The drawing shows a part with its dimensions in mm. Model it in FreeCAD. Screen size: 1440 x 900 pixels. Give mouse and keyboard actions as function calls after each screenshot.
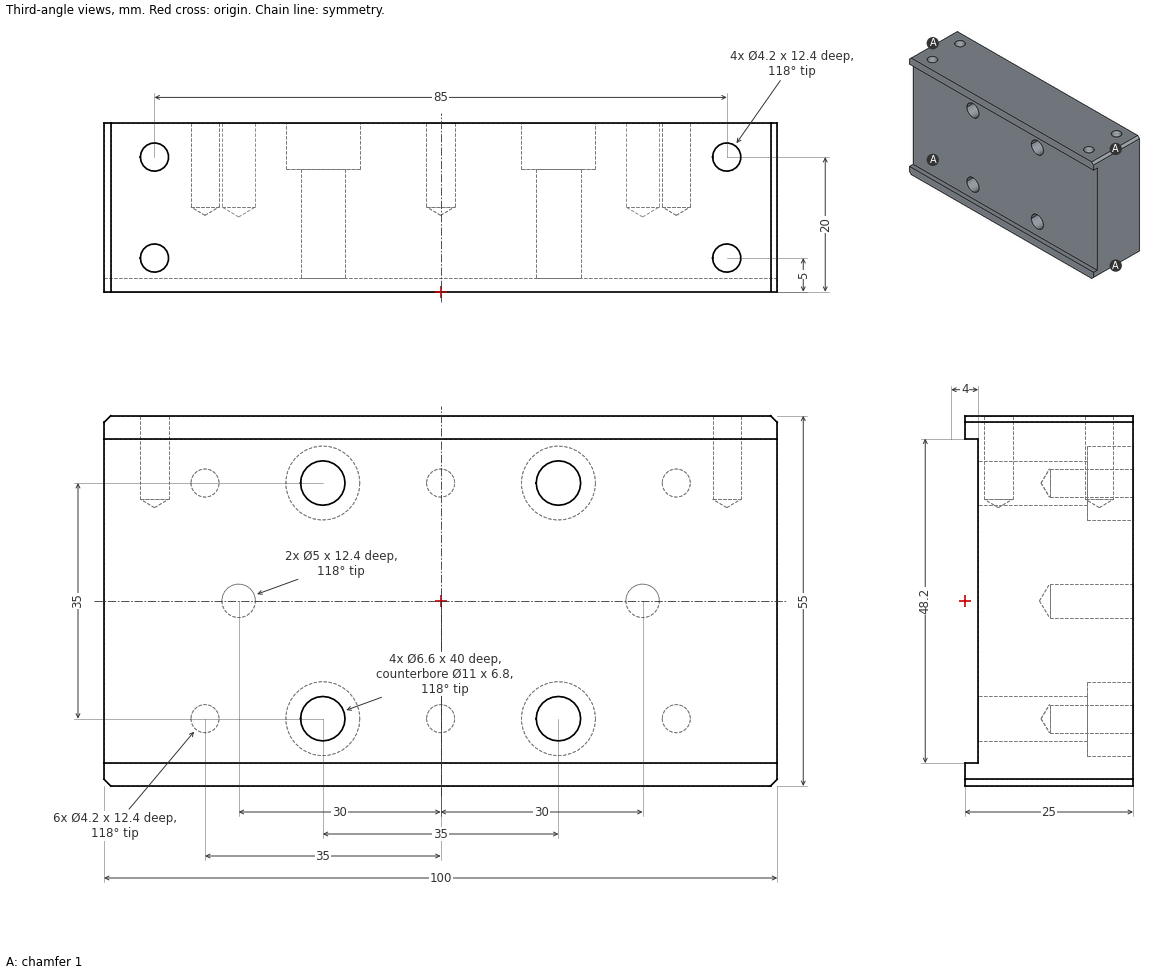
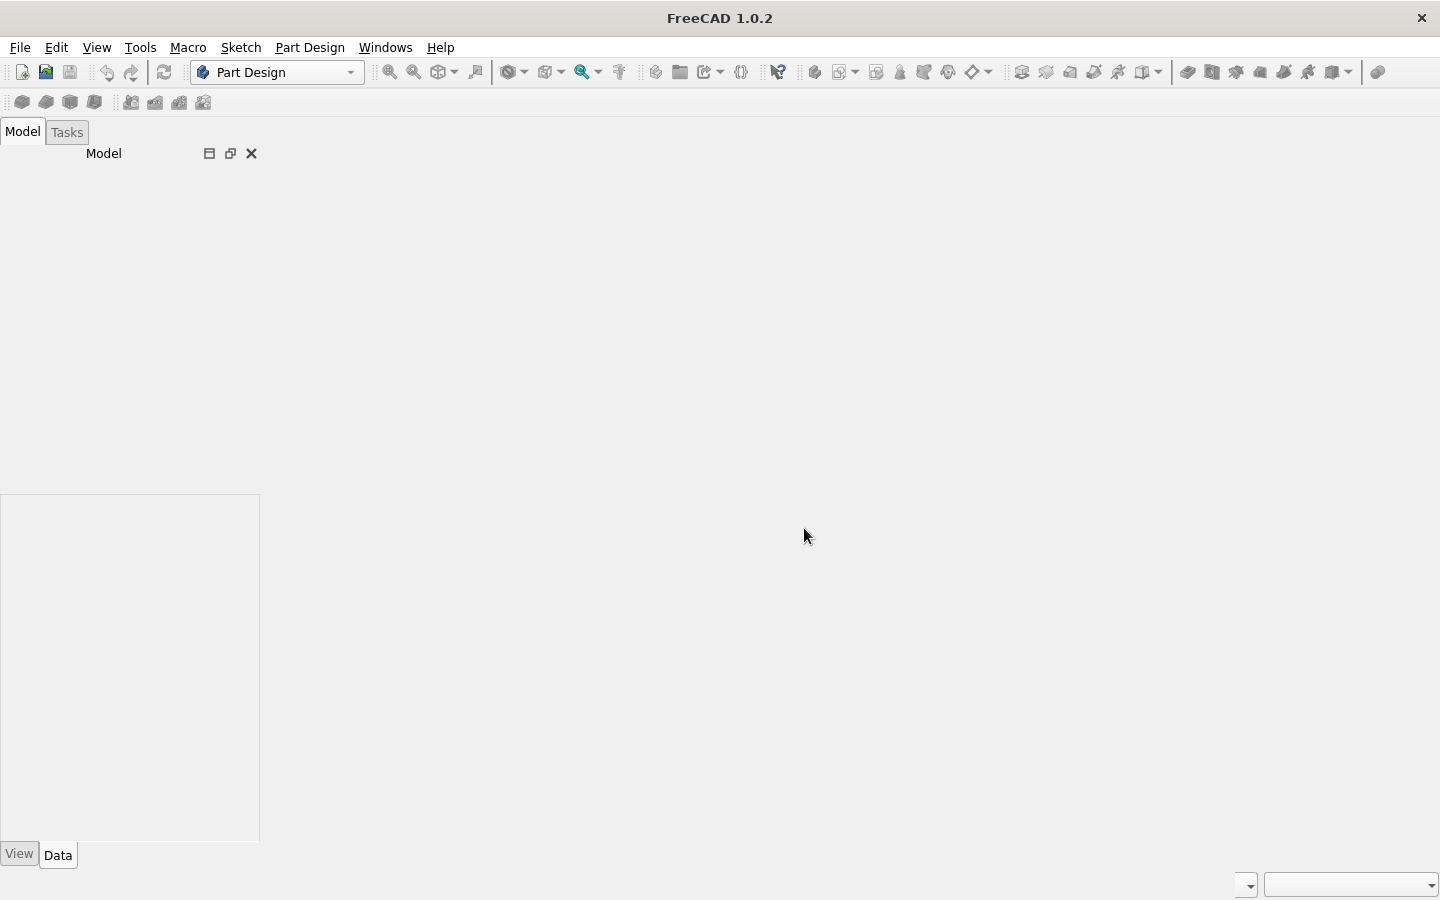
click(22, 72)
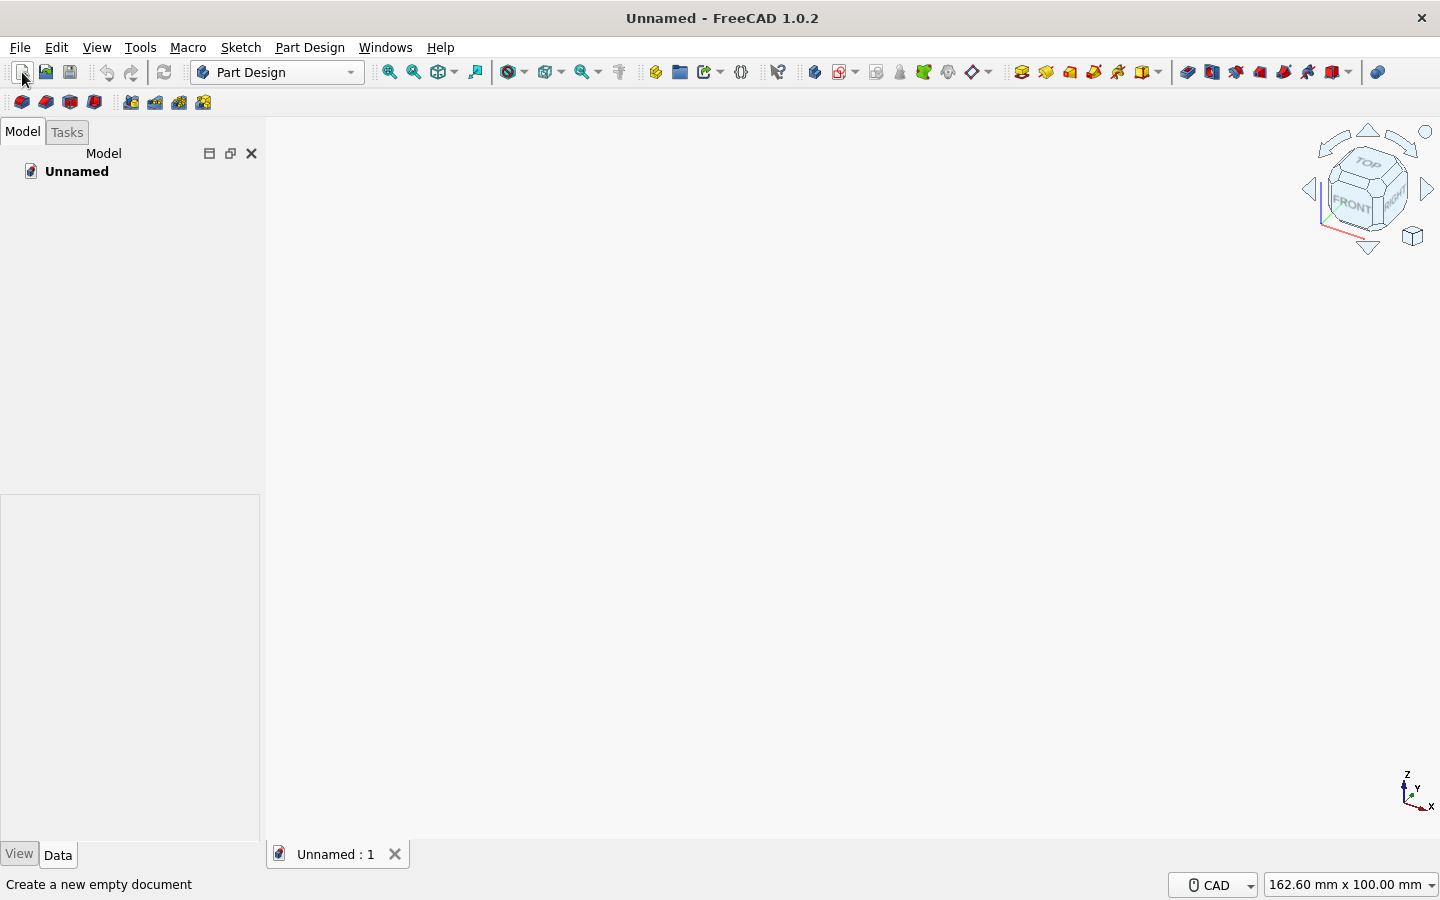
click(840, 72)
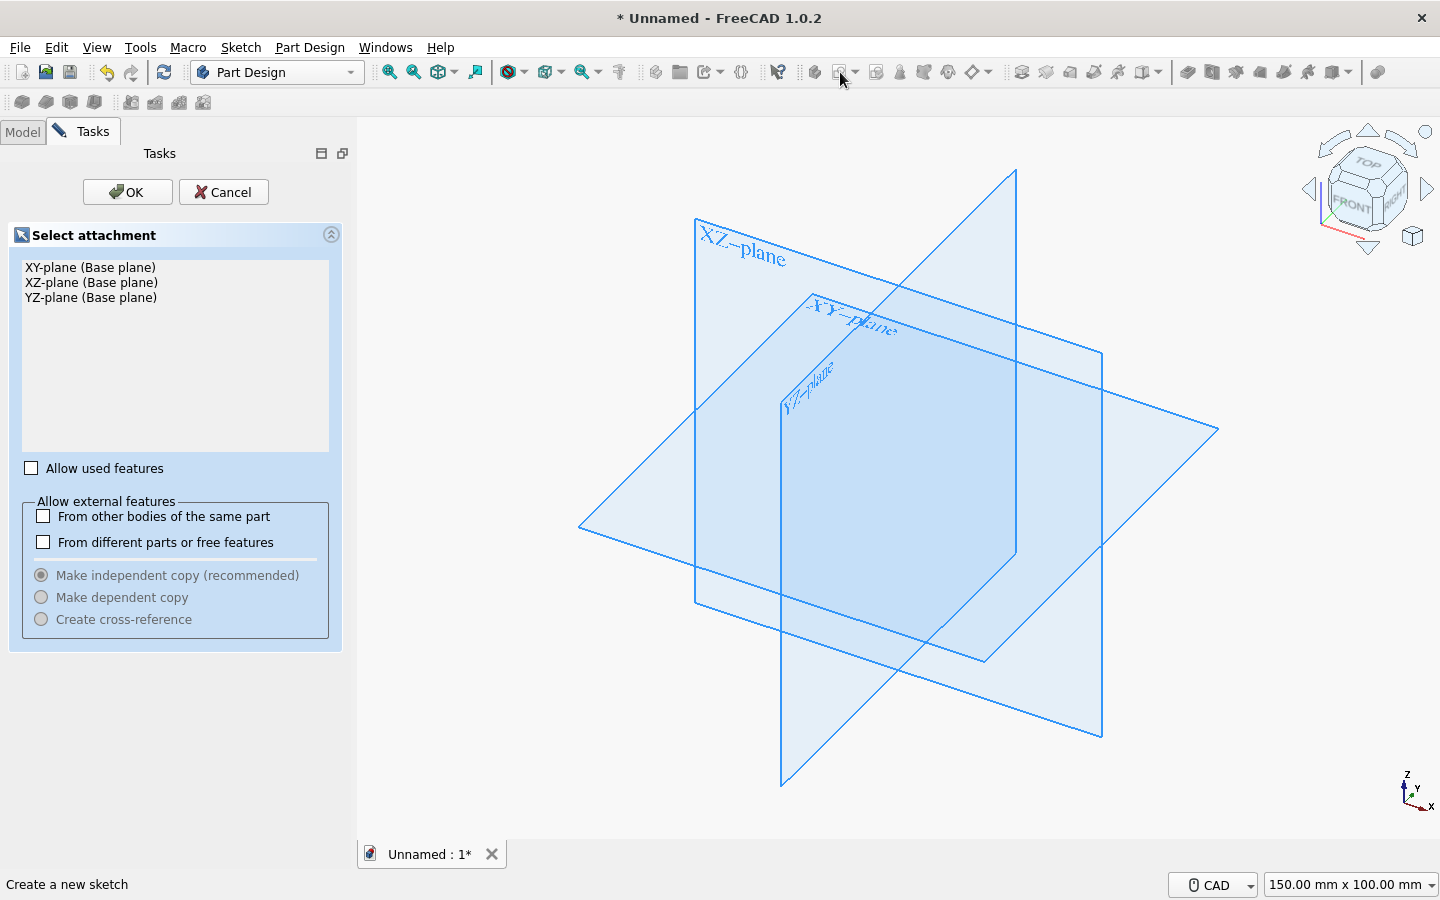
click(82, 282)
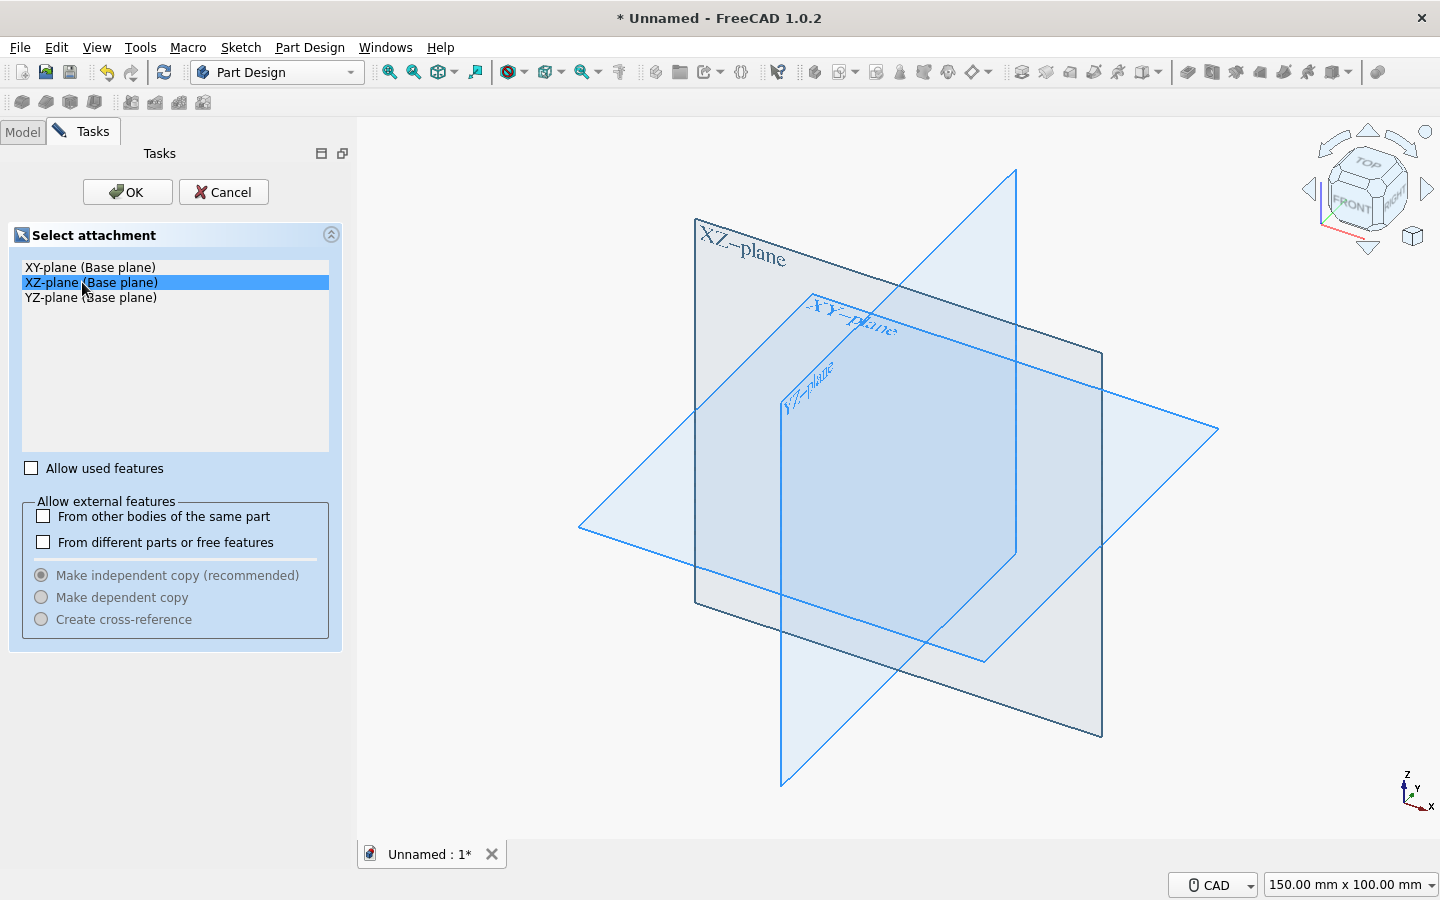
click(128, 192)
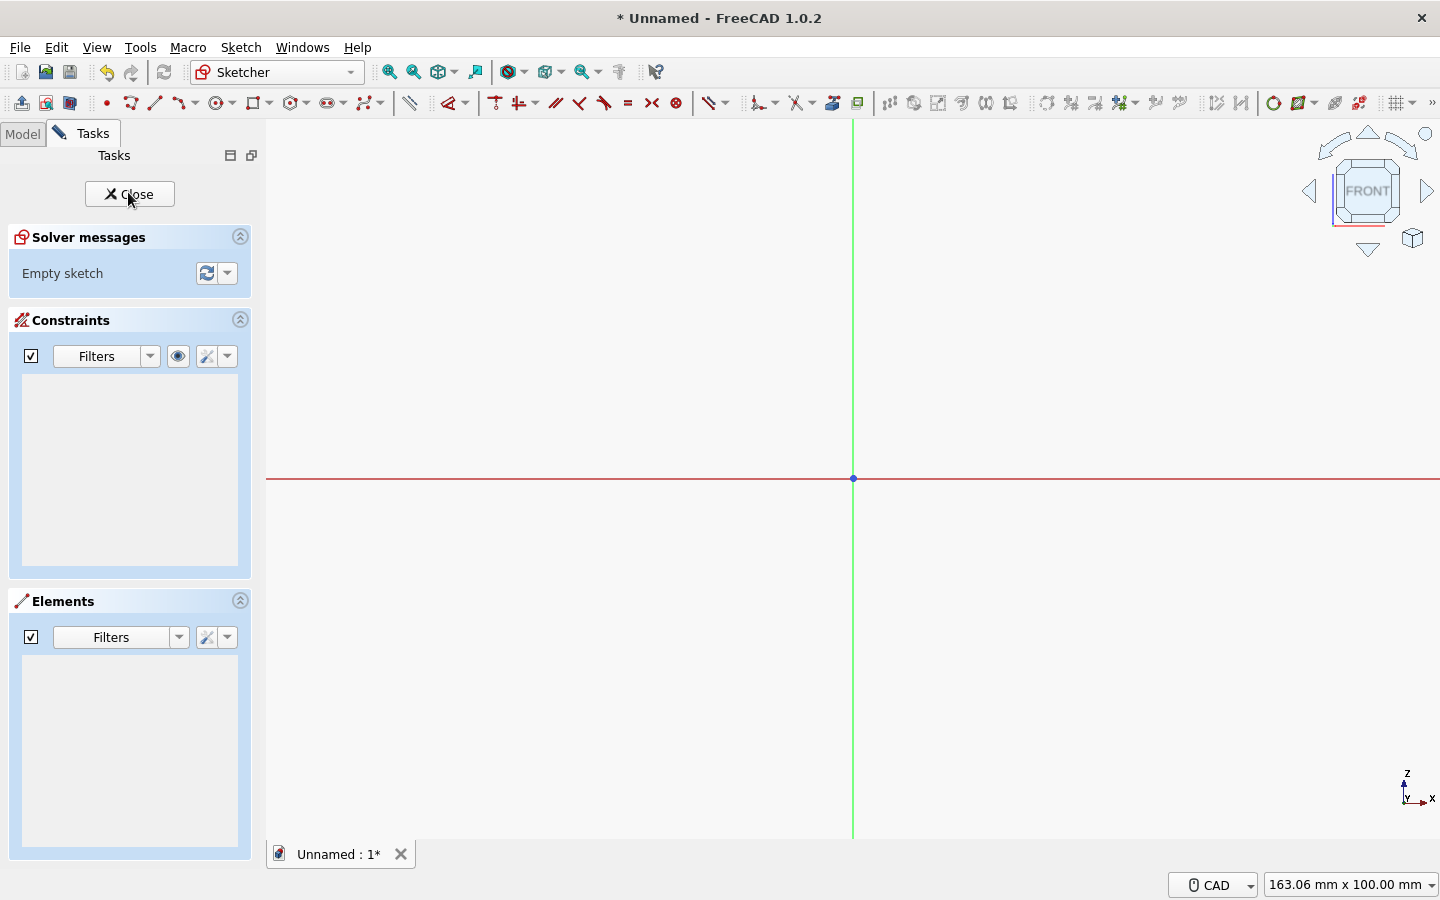
click(272, 104)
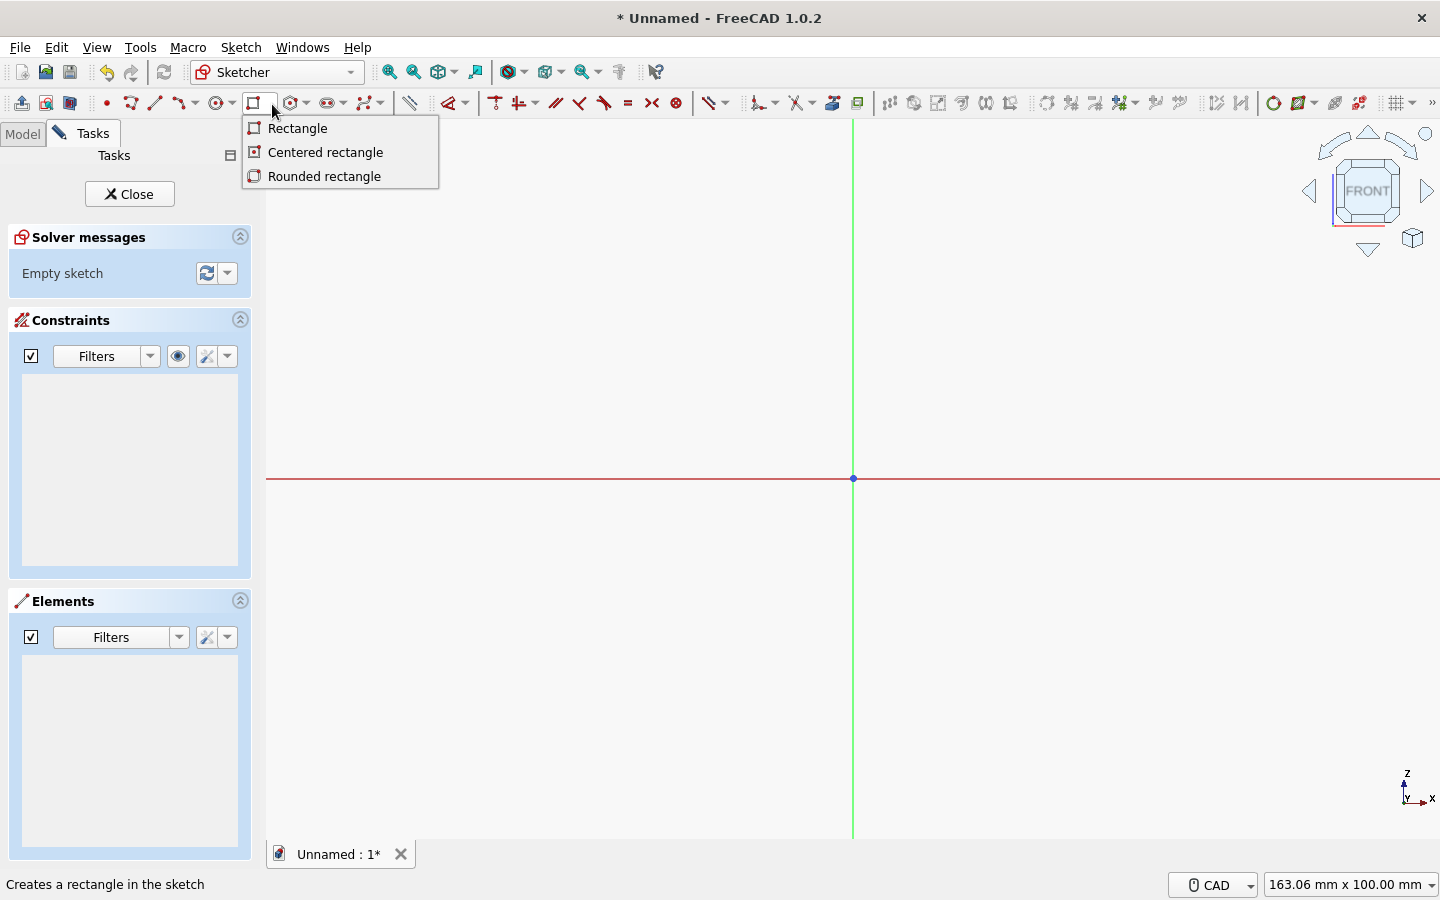
click(340, 152)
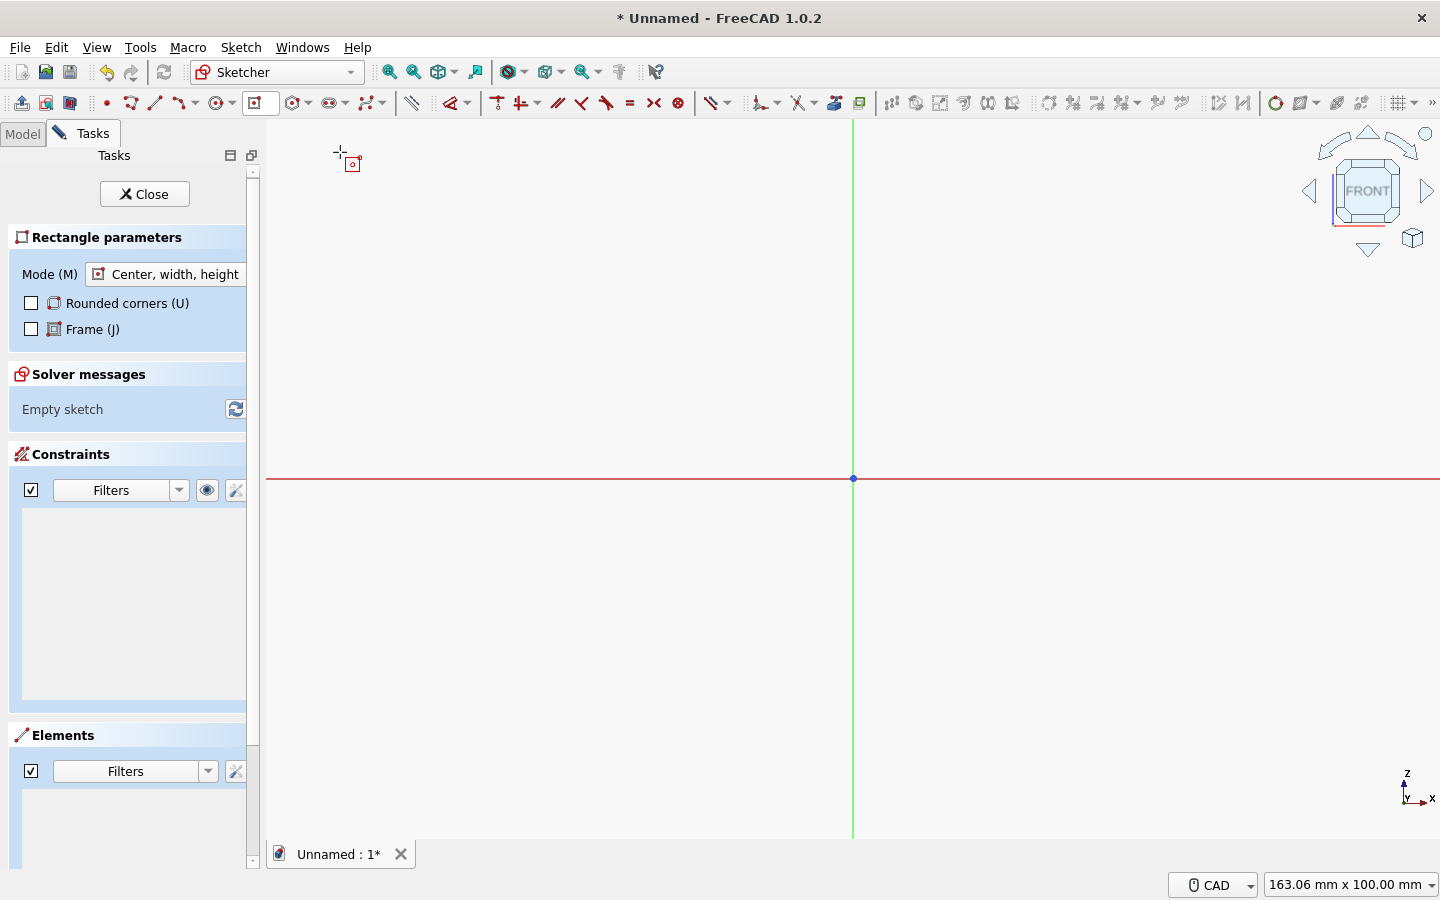
click(853, 479)
move(1213, 281)